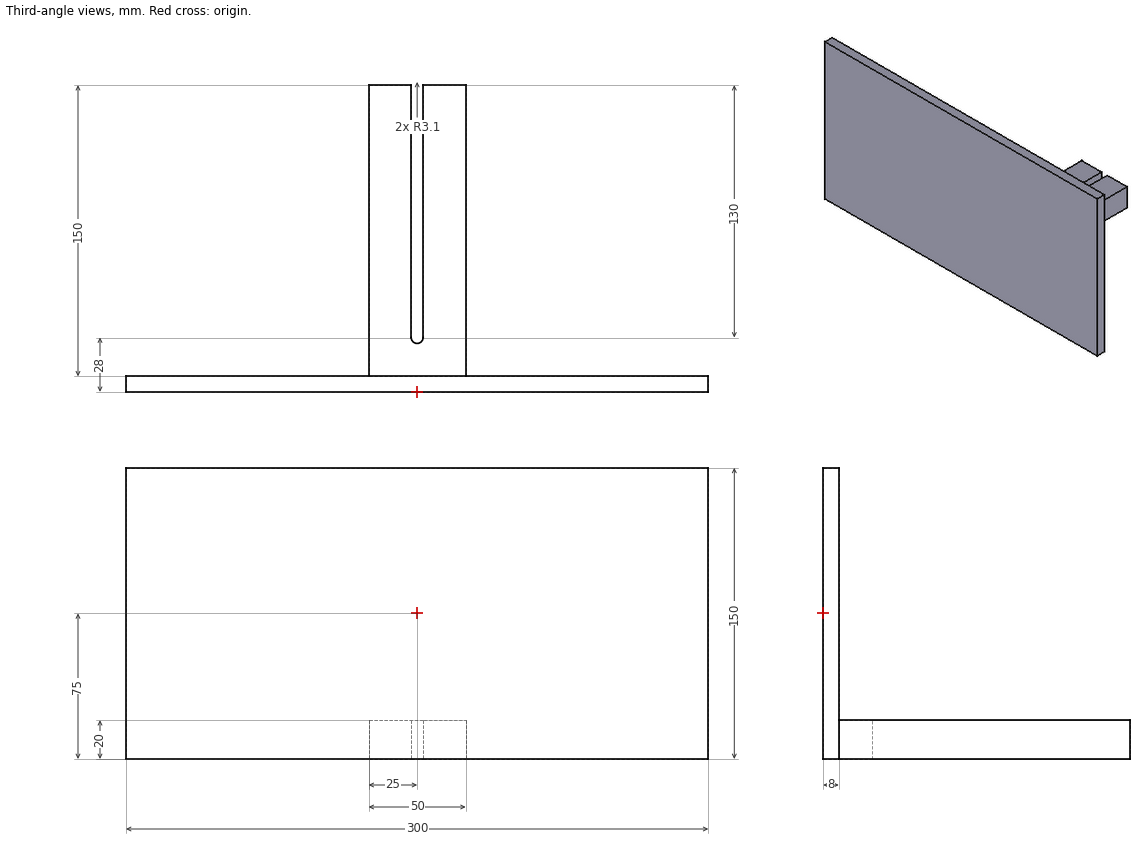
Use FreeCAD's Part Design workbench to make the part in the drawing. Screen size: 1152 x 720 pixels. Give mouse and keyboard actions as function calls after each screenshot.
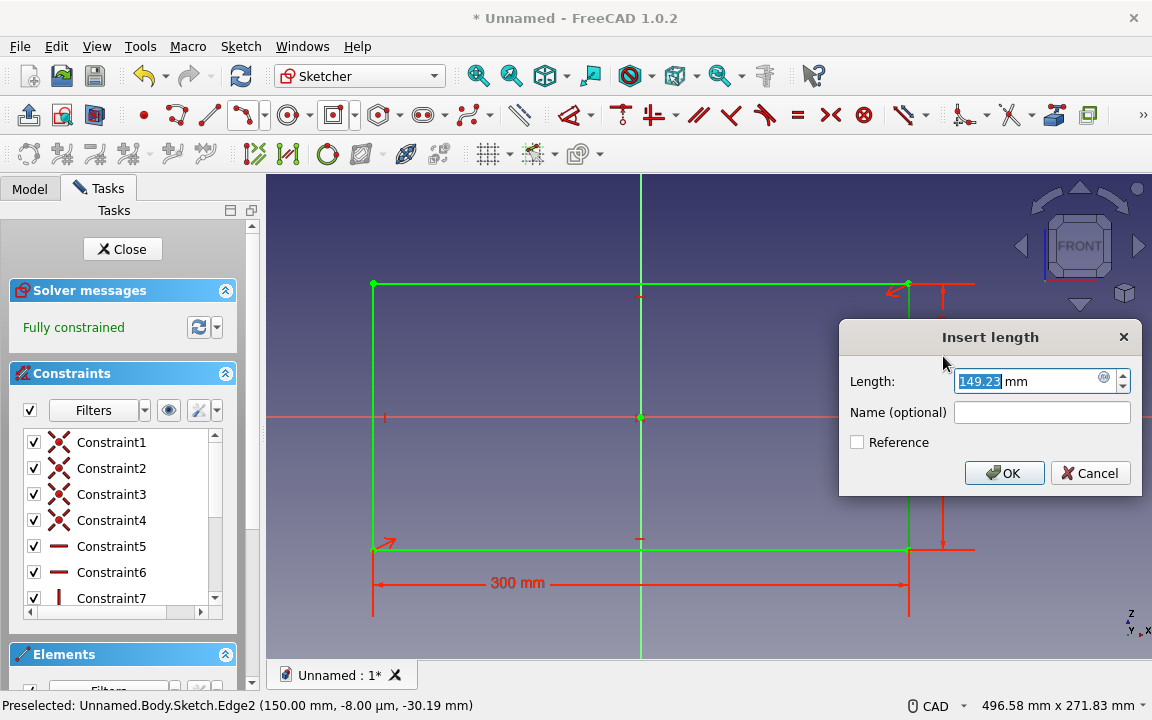
text(150)
key(Return)
key(Escape)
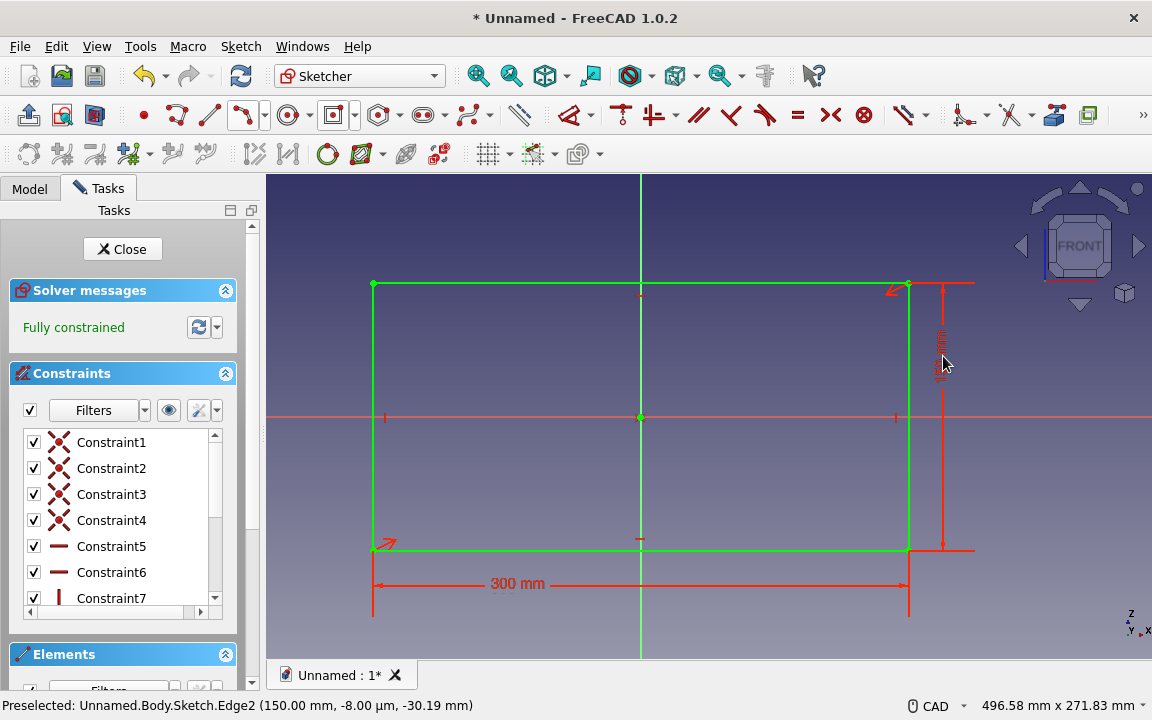
click(123, 249)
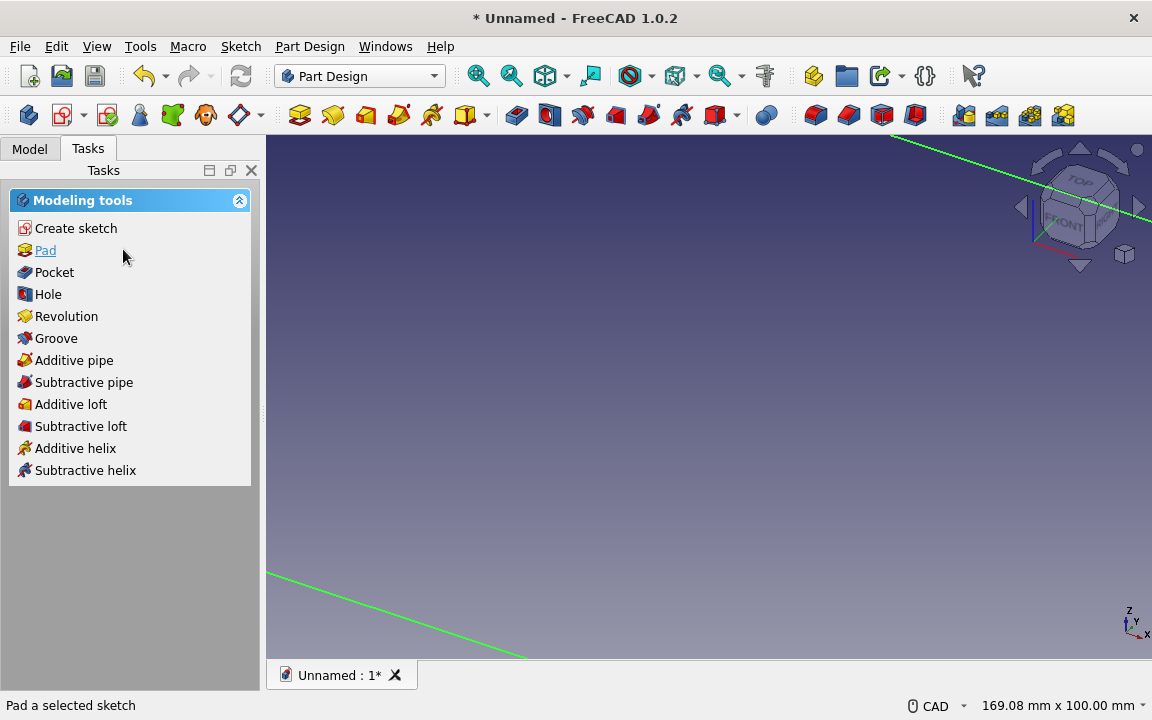
click(300, 116)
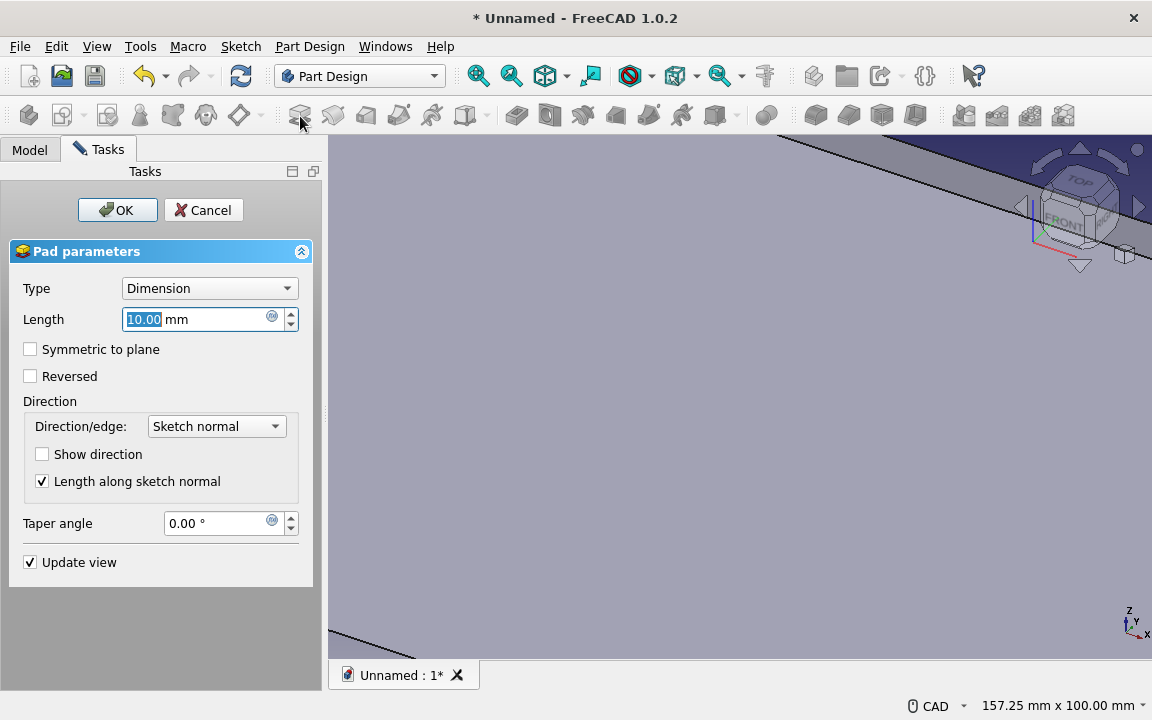
text(8)
key(Tab)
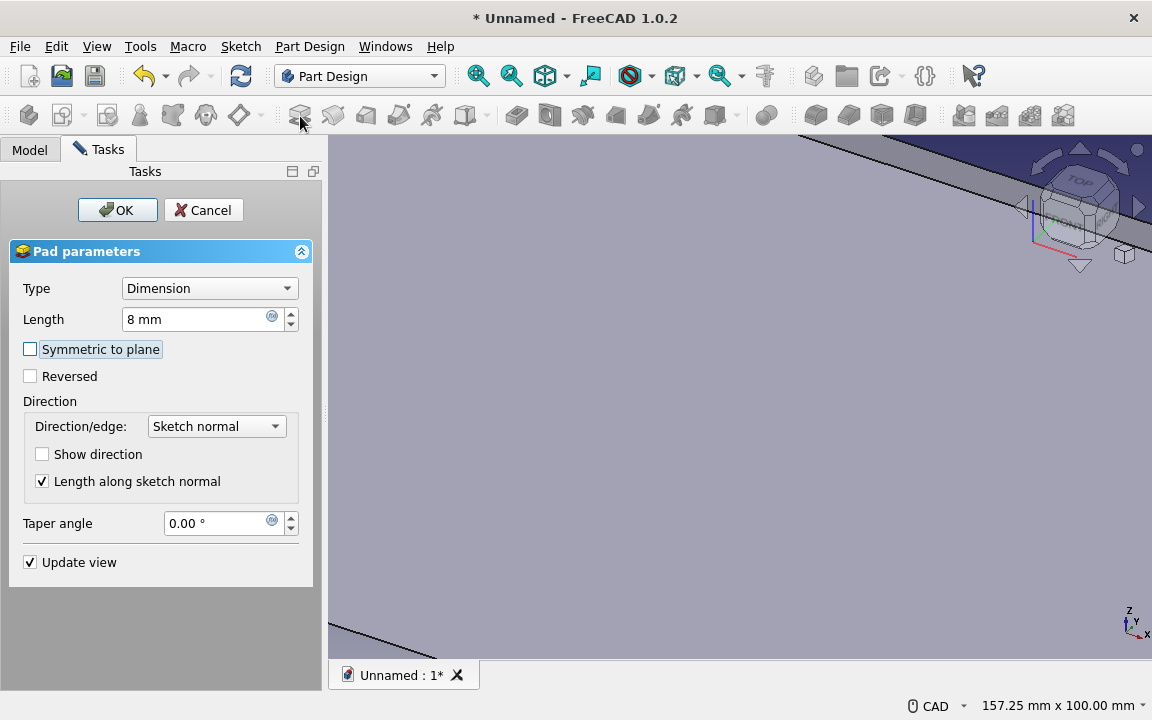
click(31, 376)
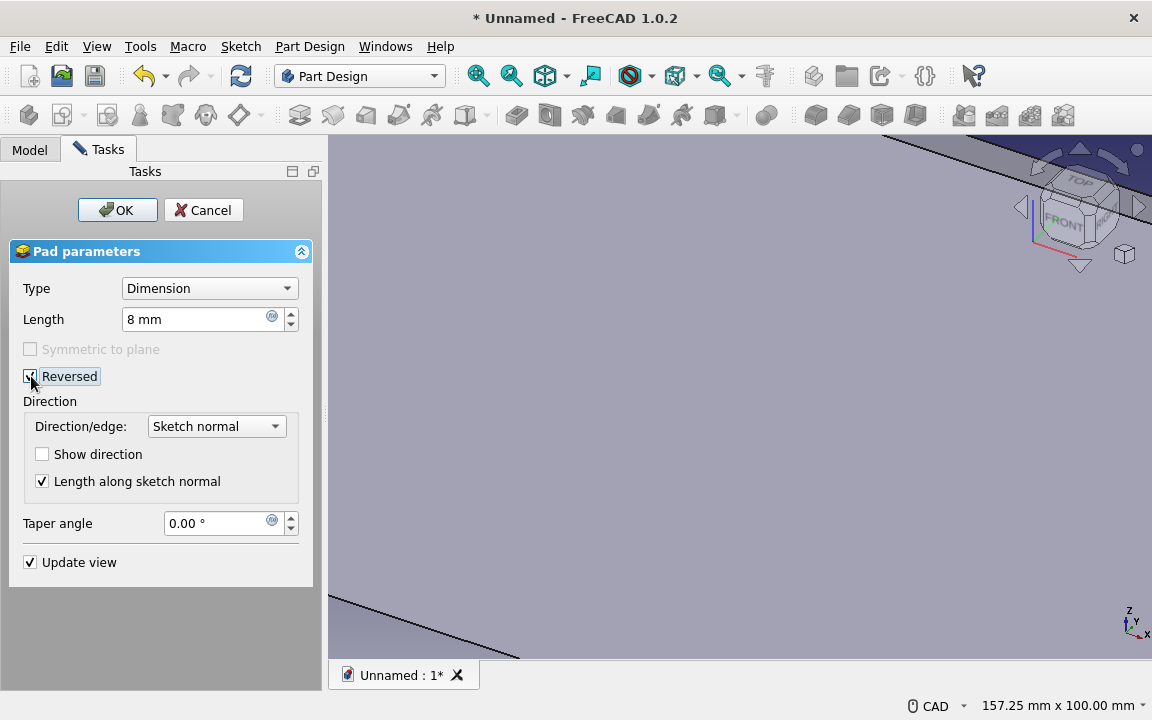
click(118, 210)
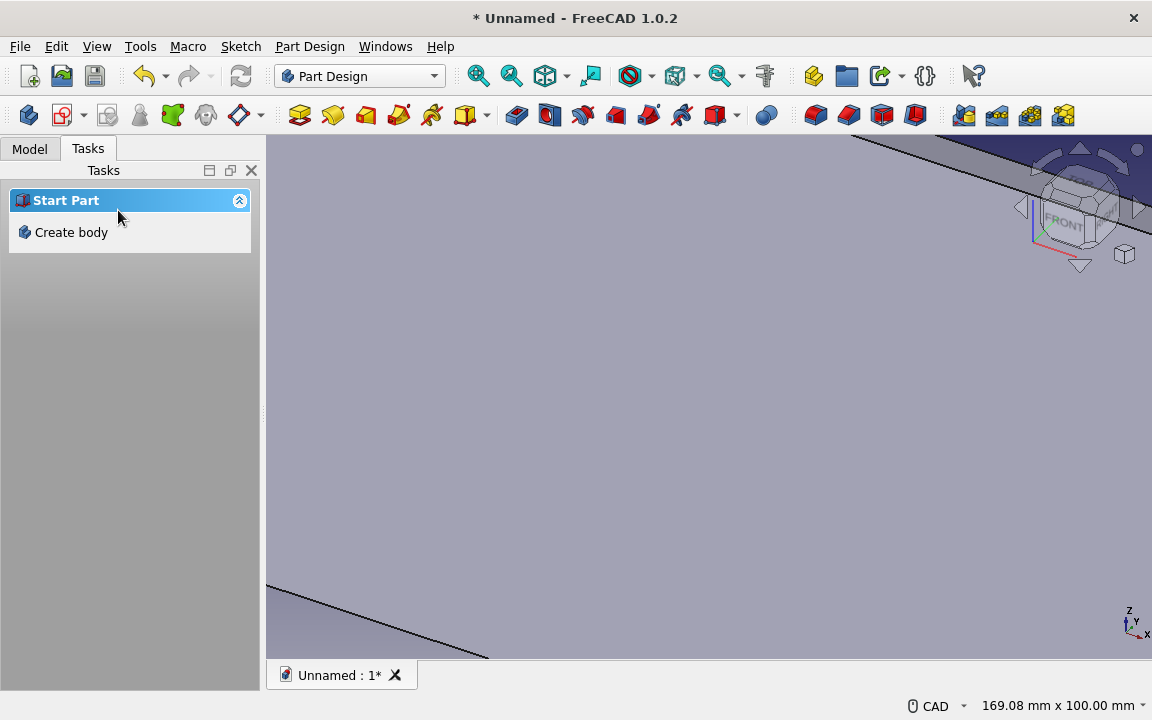
click(479, 76)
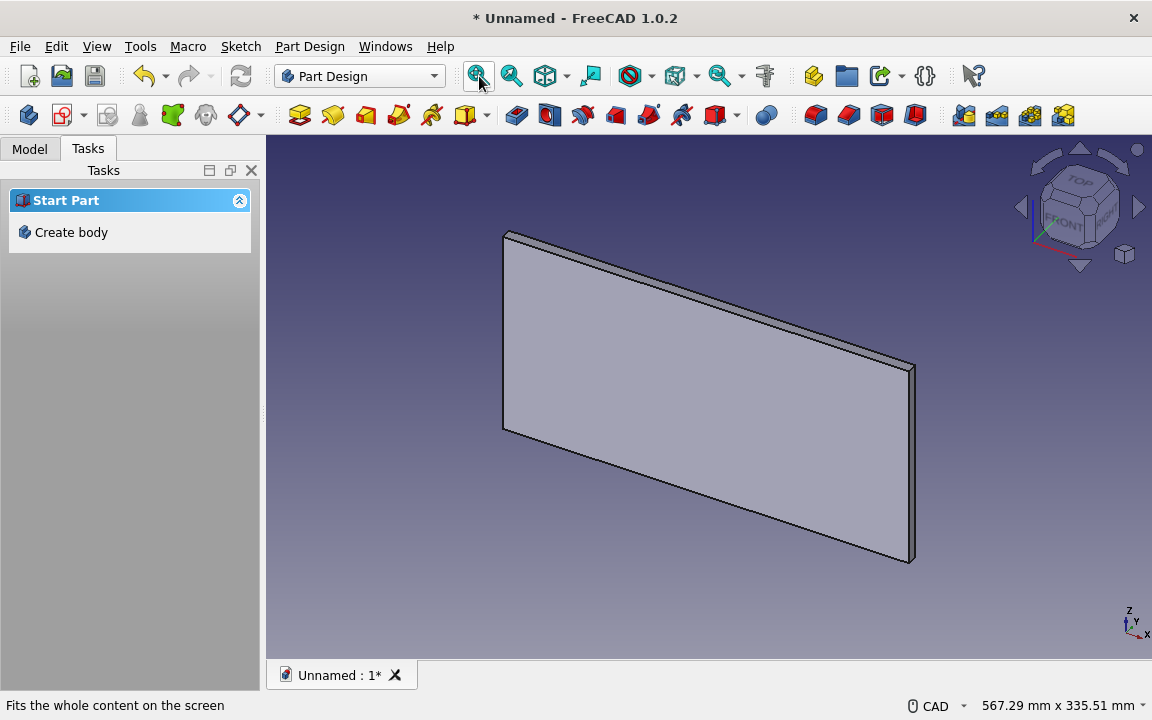
key(4)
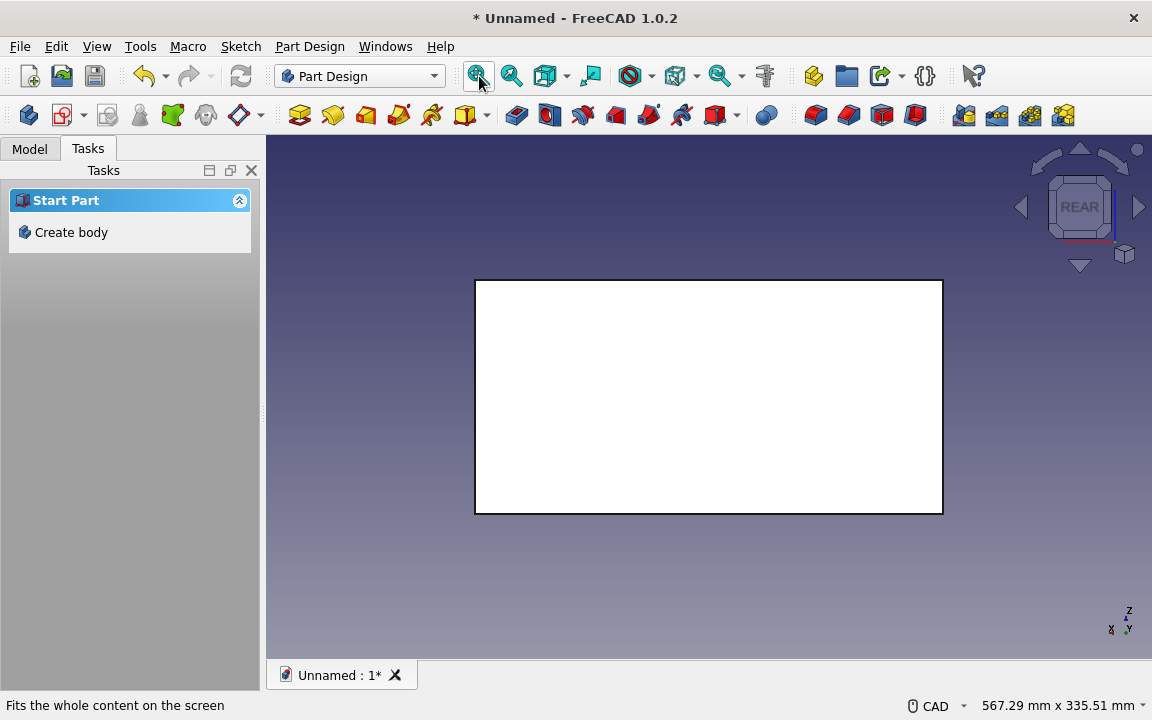
click(642, 396)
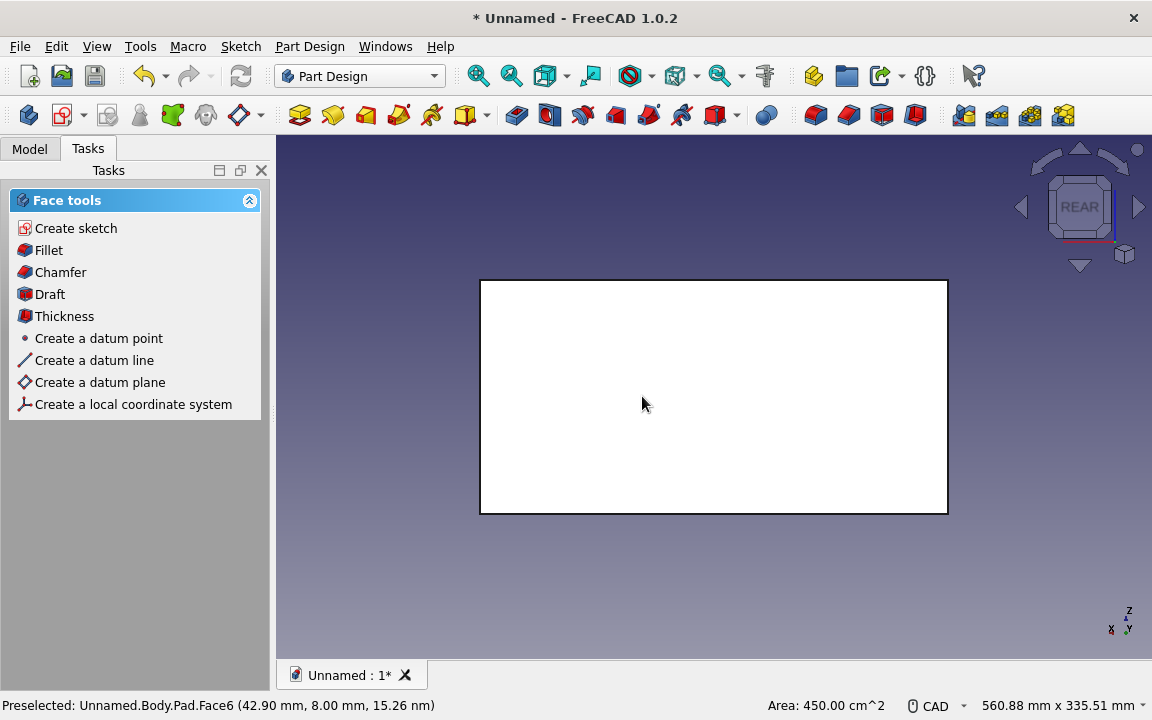
click(62, 116)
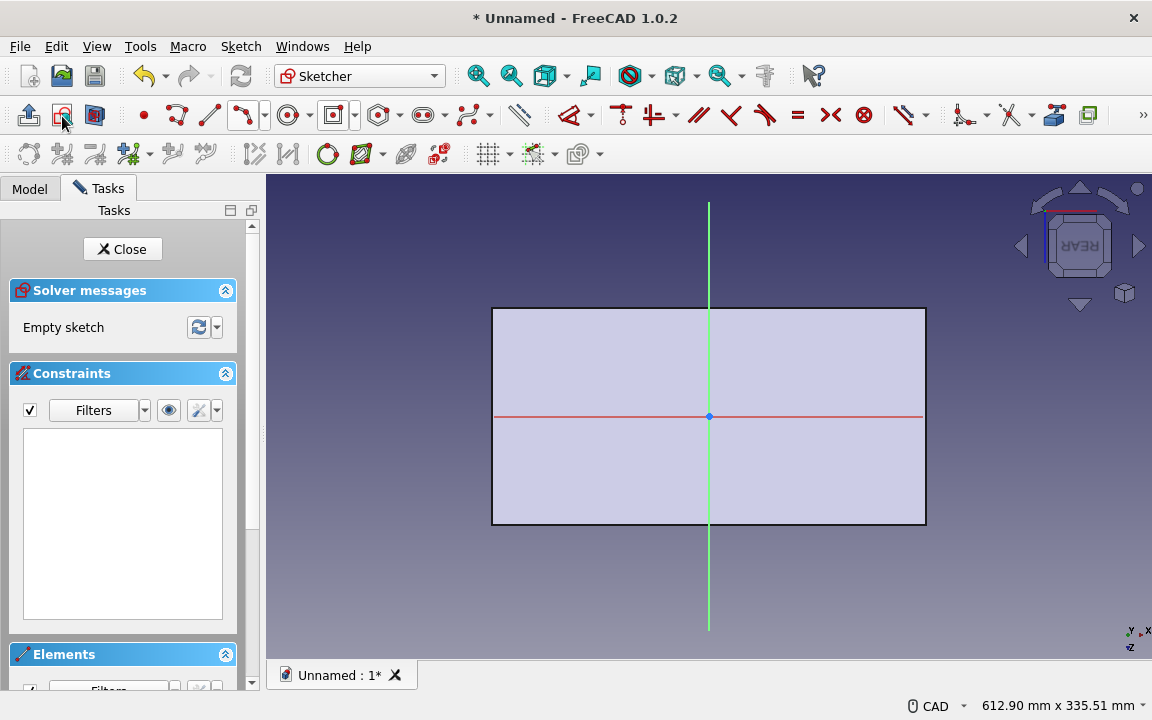
scroll(749, 331, up, 5)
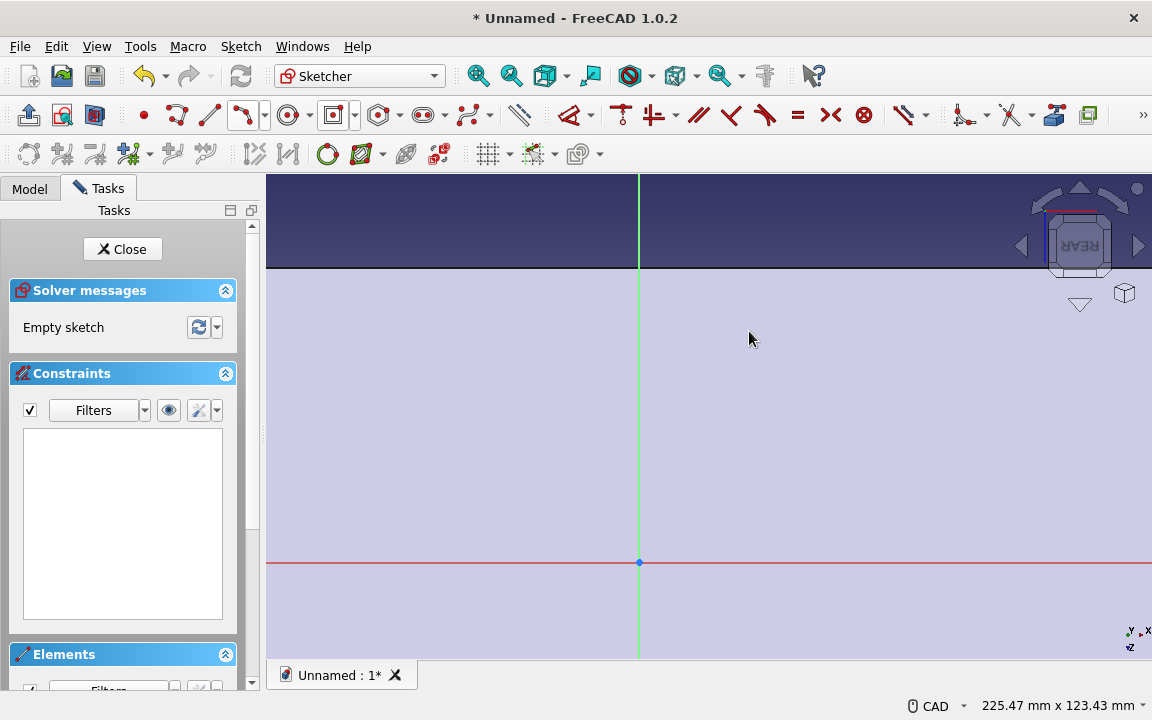
click(354, 116)